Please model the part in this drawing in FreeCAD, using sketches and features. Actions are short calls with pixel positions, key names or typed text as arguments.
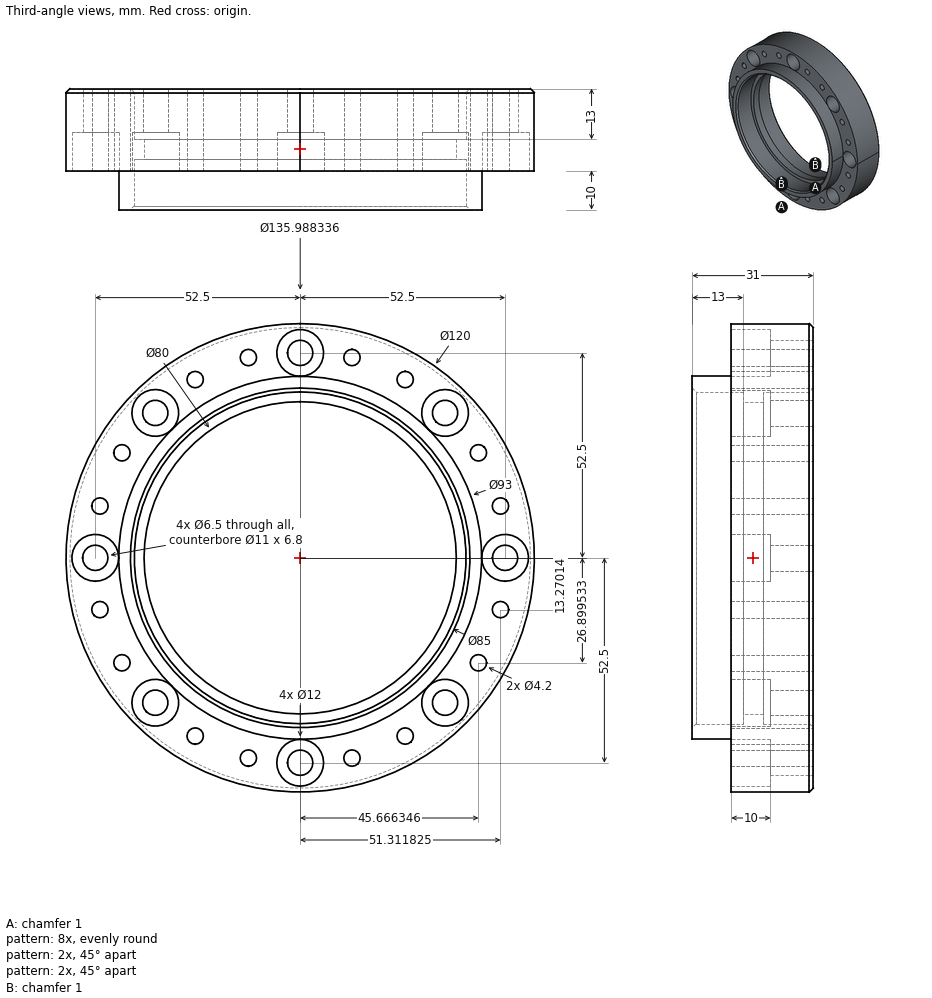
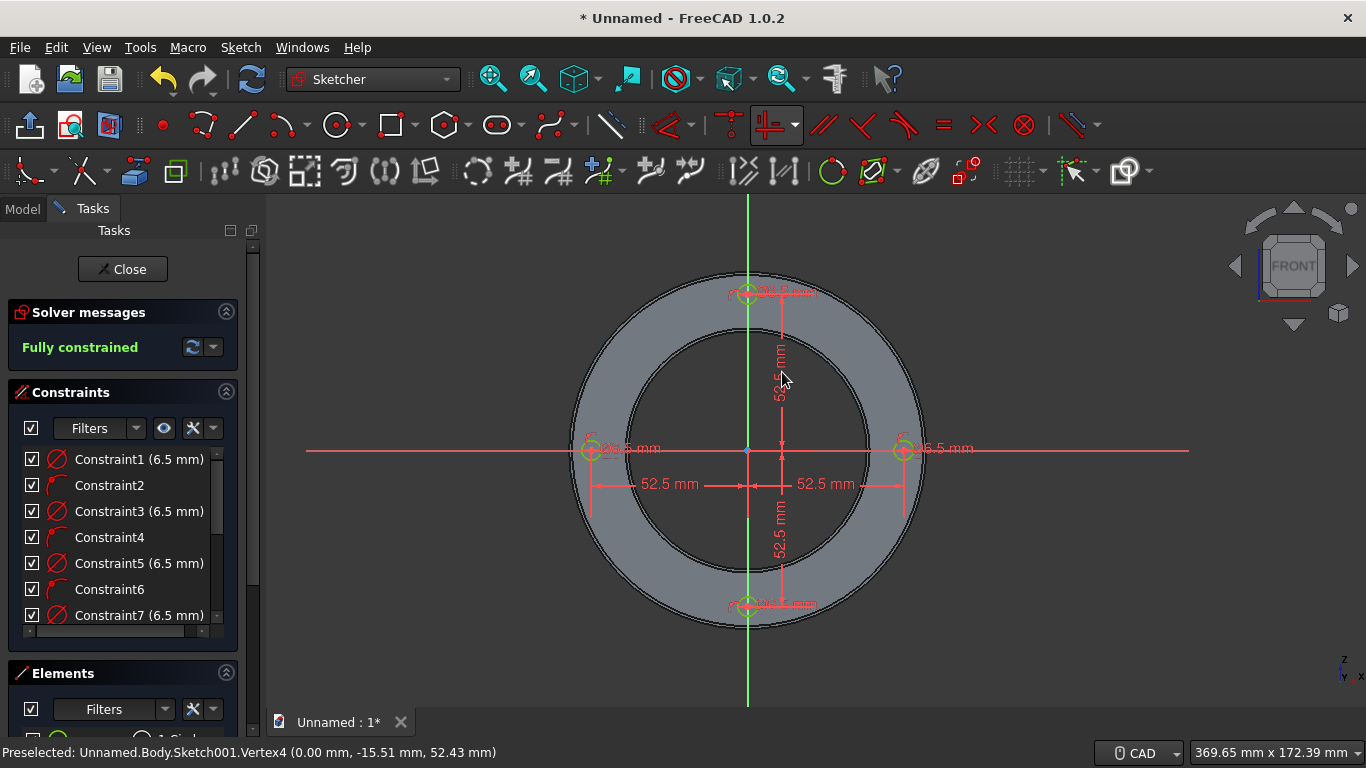
click(123, 269)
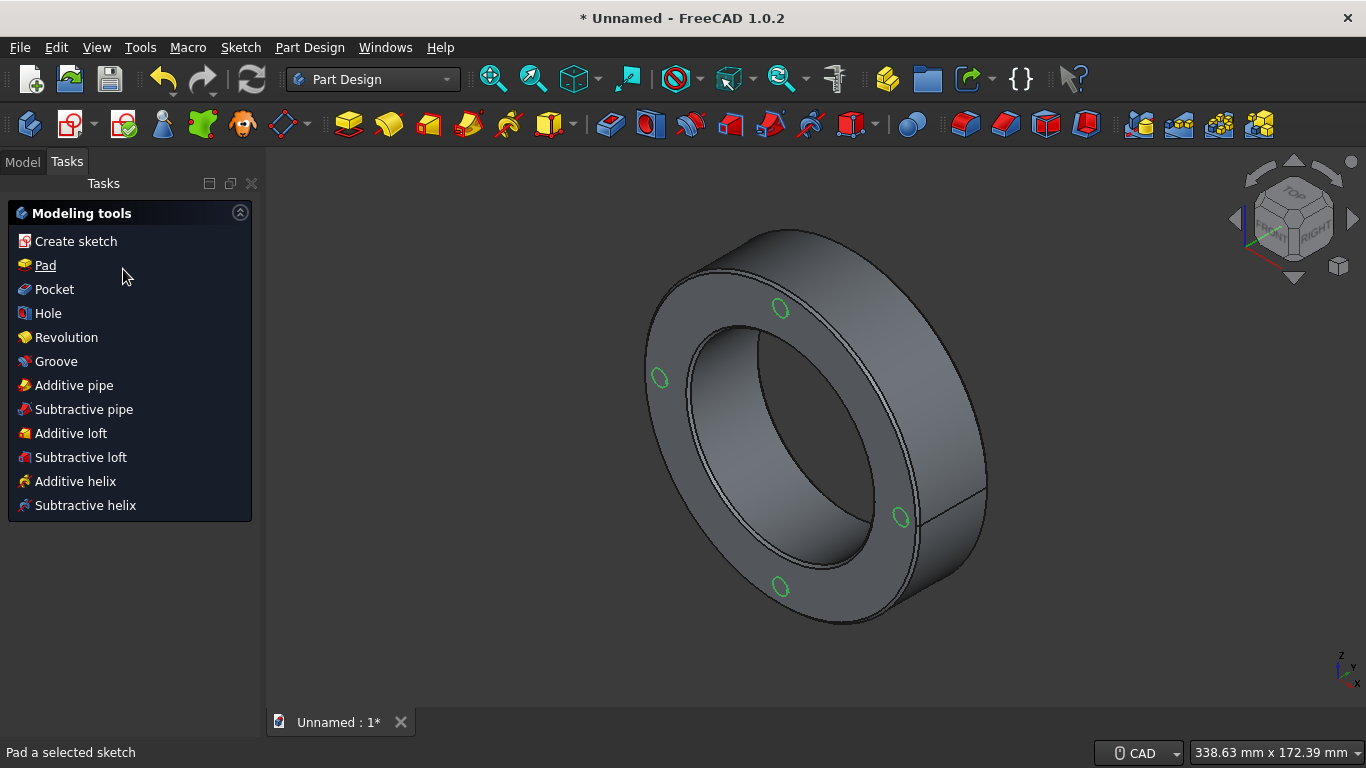
click(652, 124)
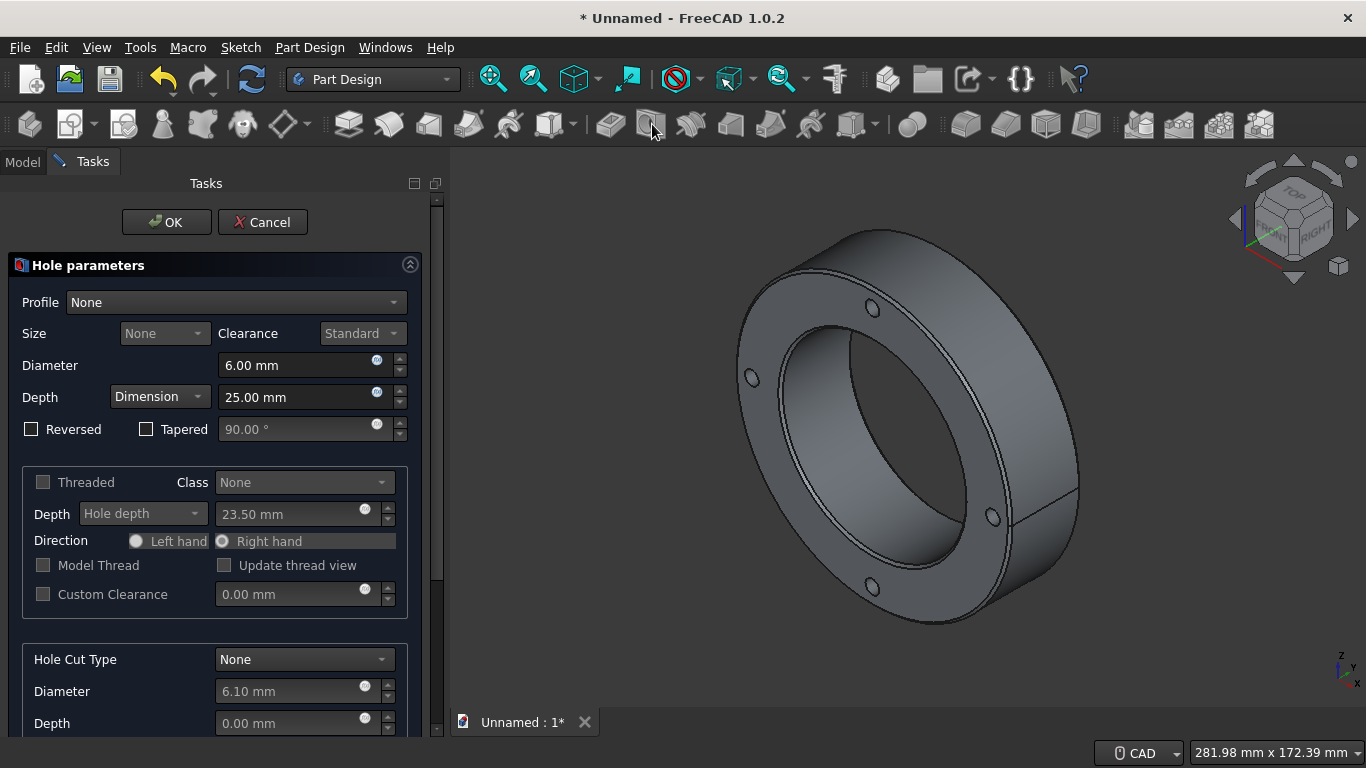
triple_click(305, 365)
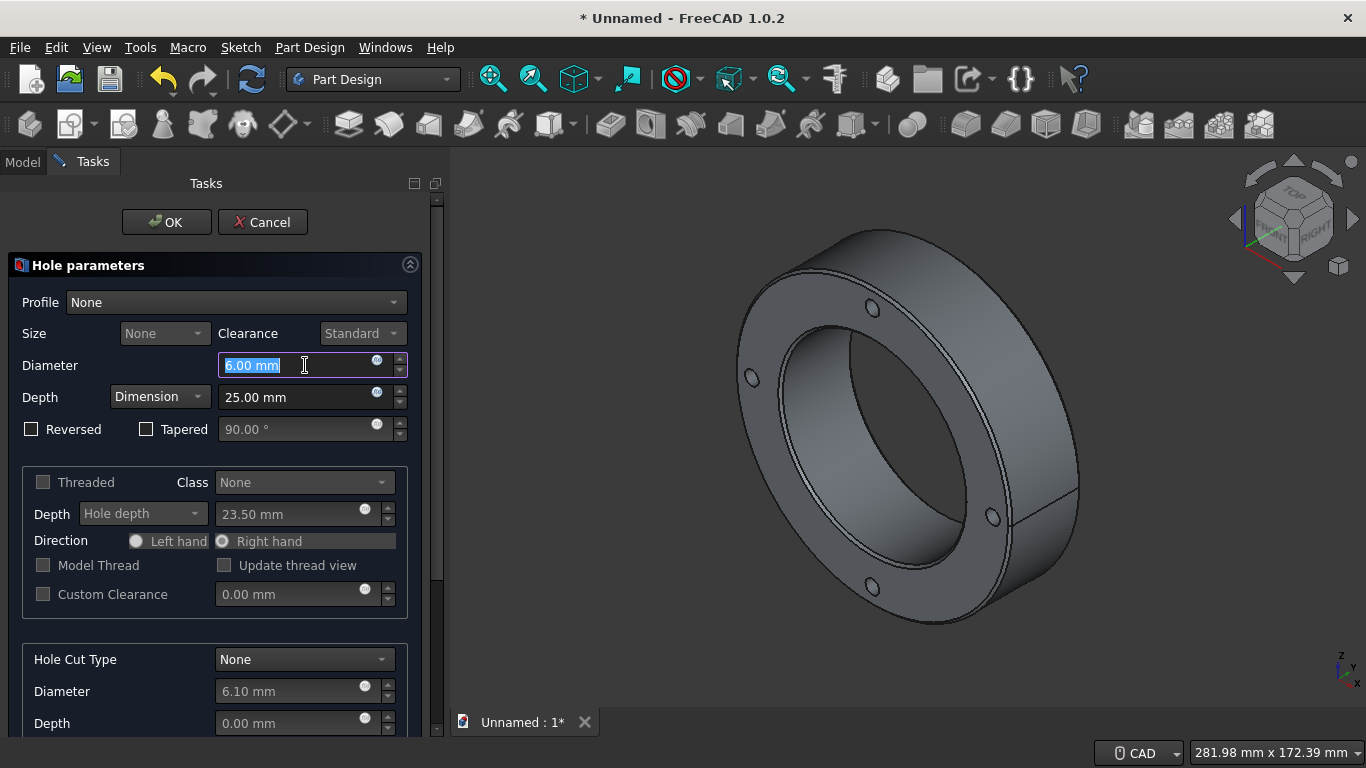
text(6.5)
key(Tab)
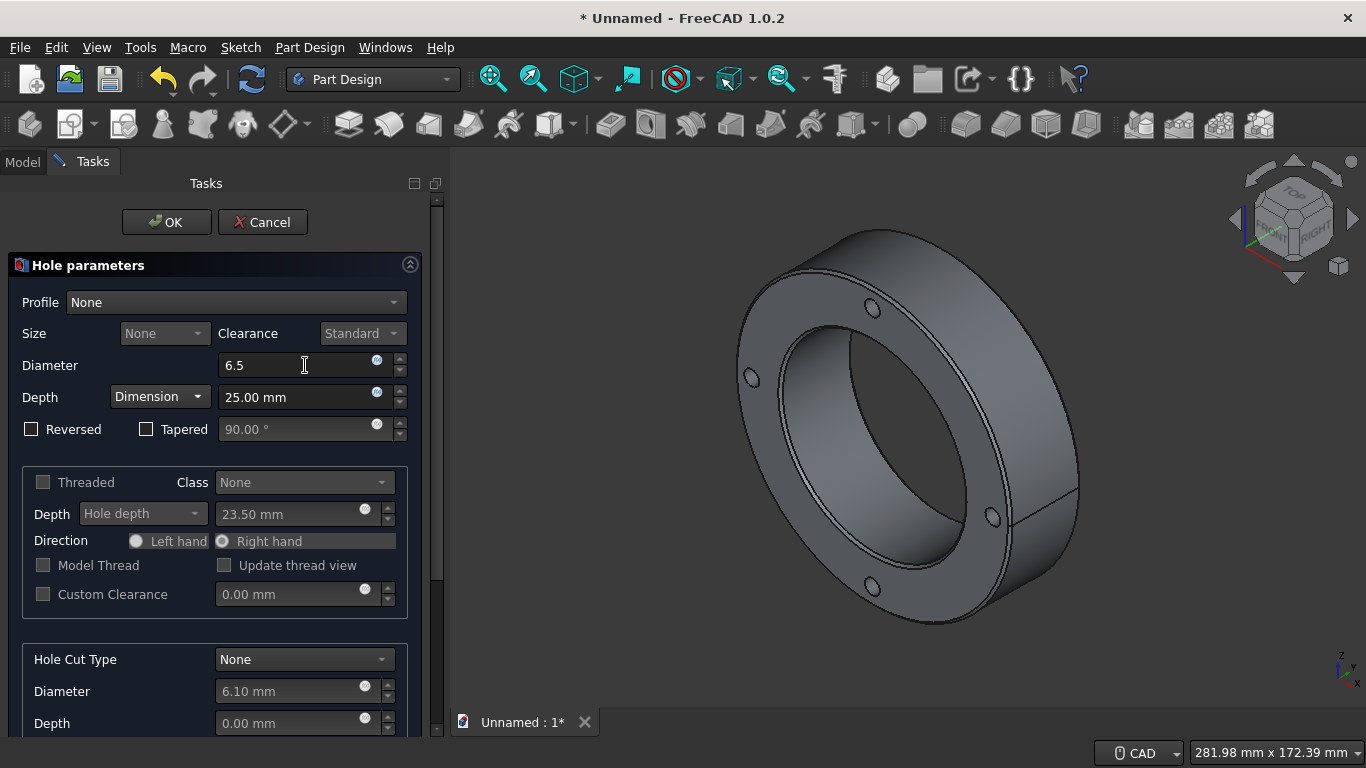
click(161, 396)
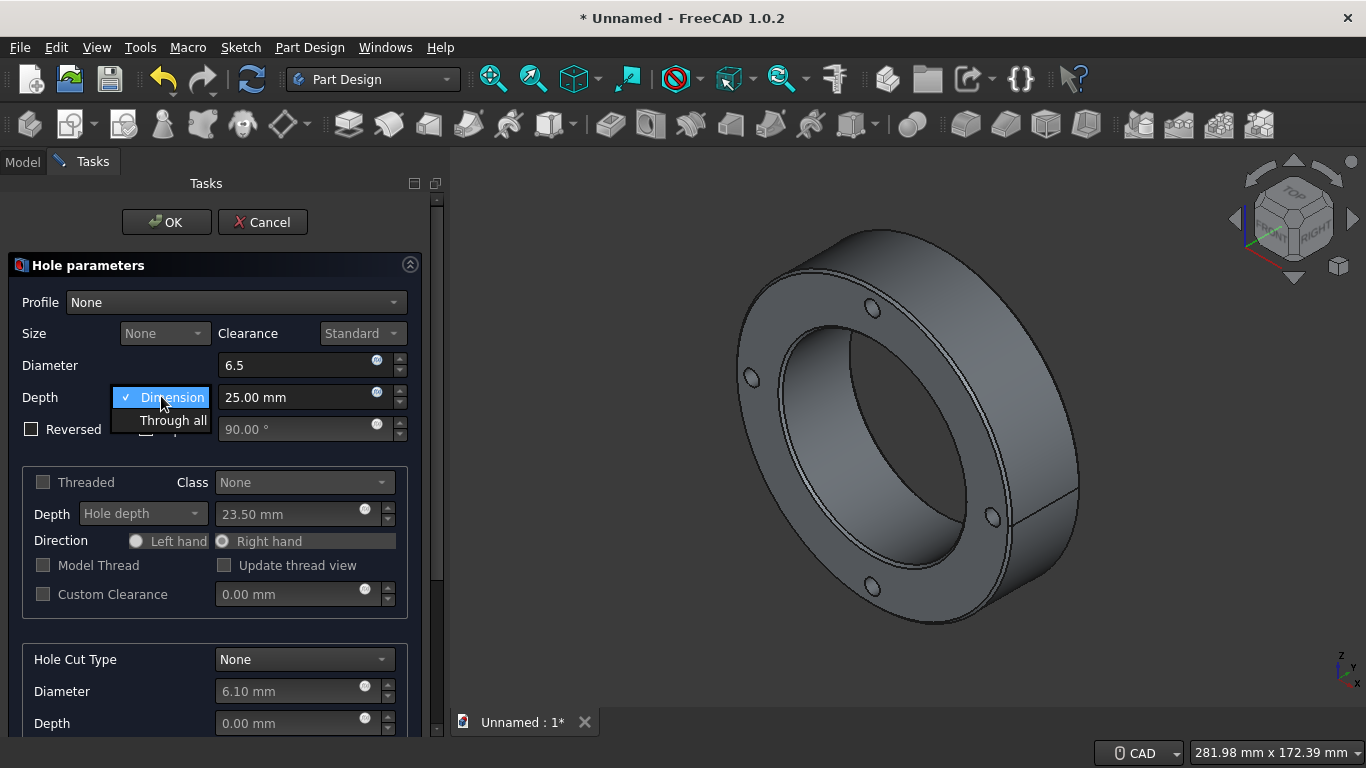
click(160, 420)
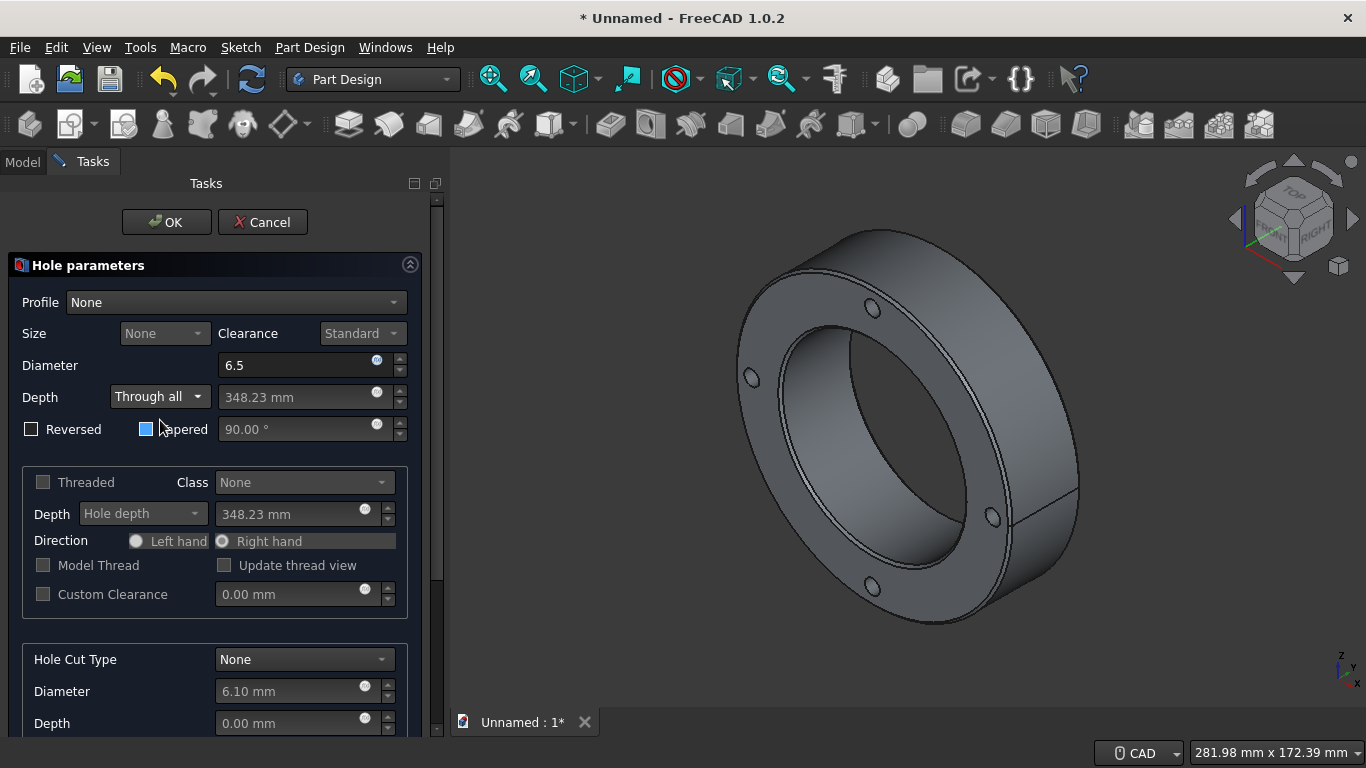
click(306, 660)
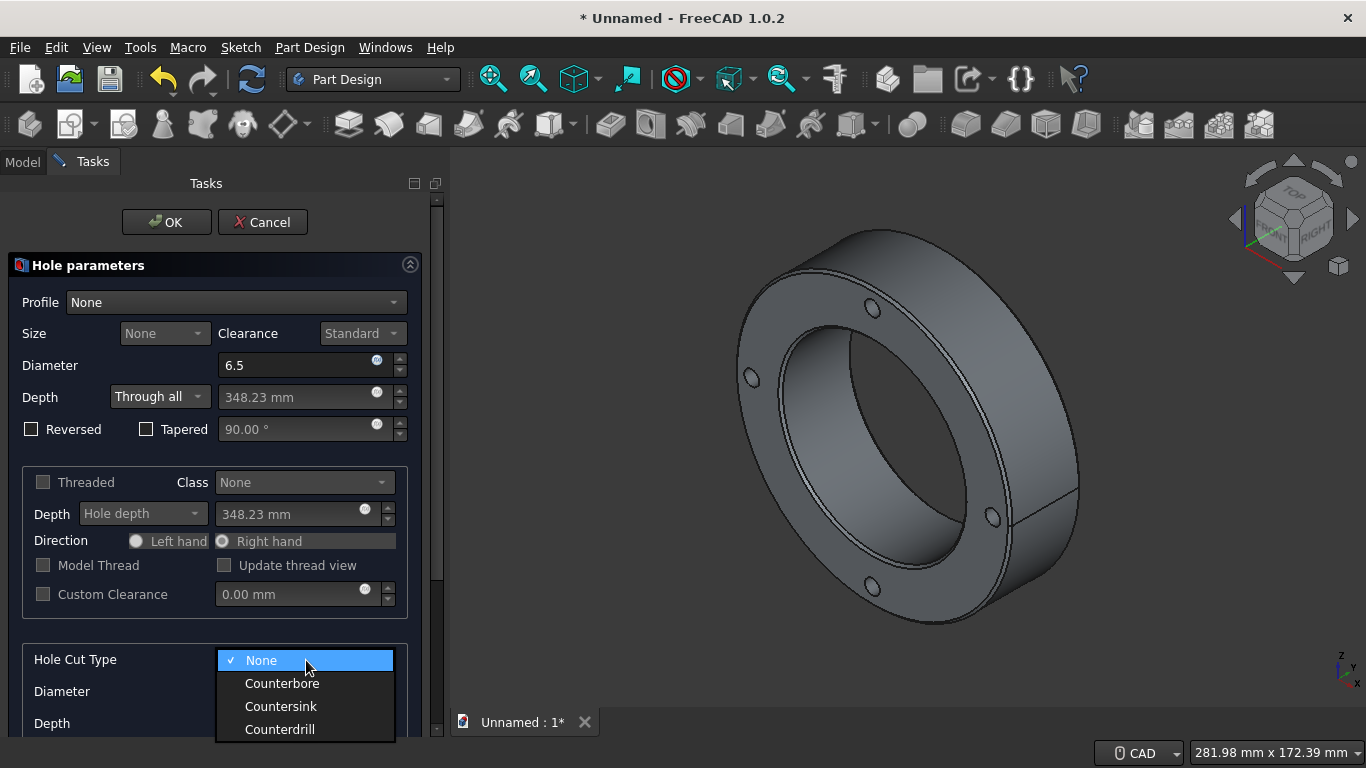
click(304, 684)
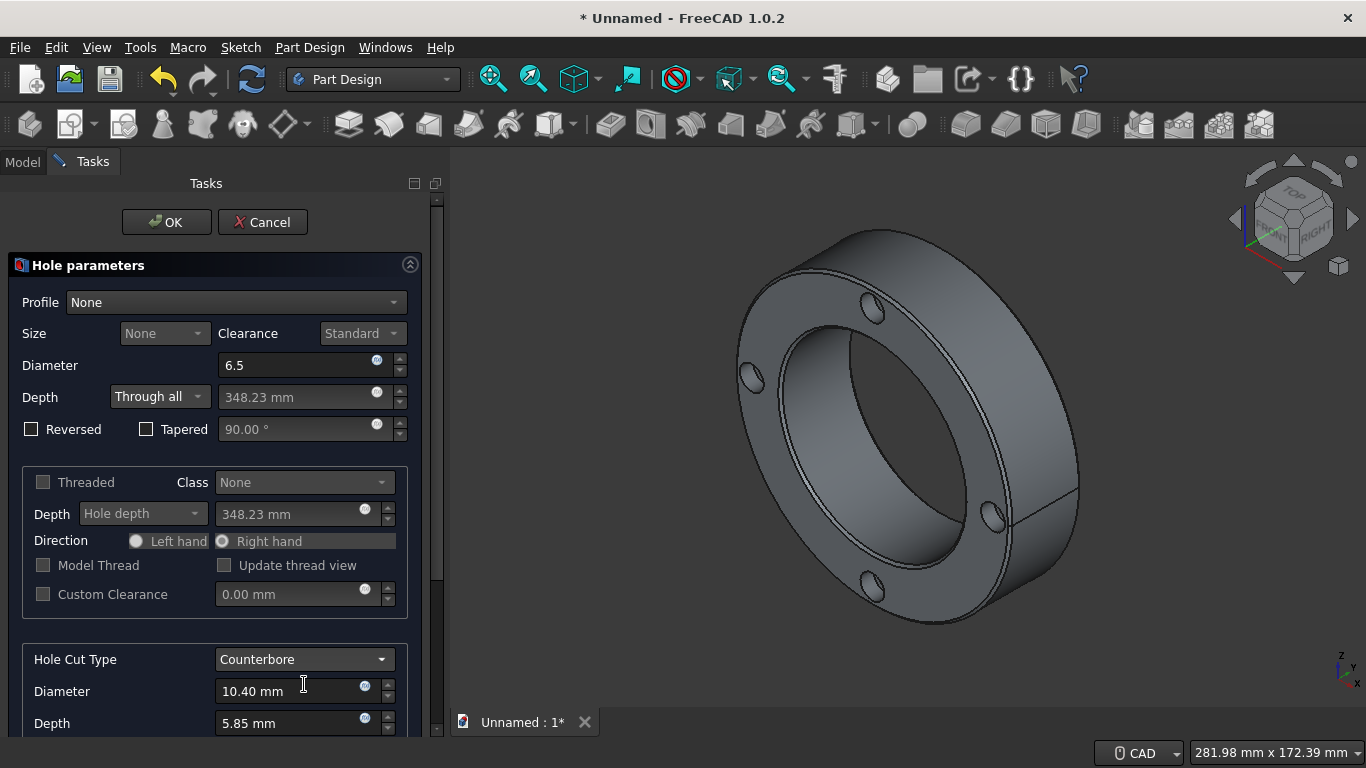
triple_click(298, 691)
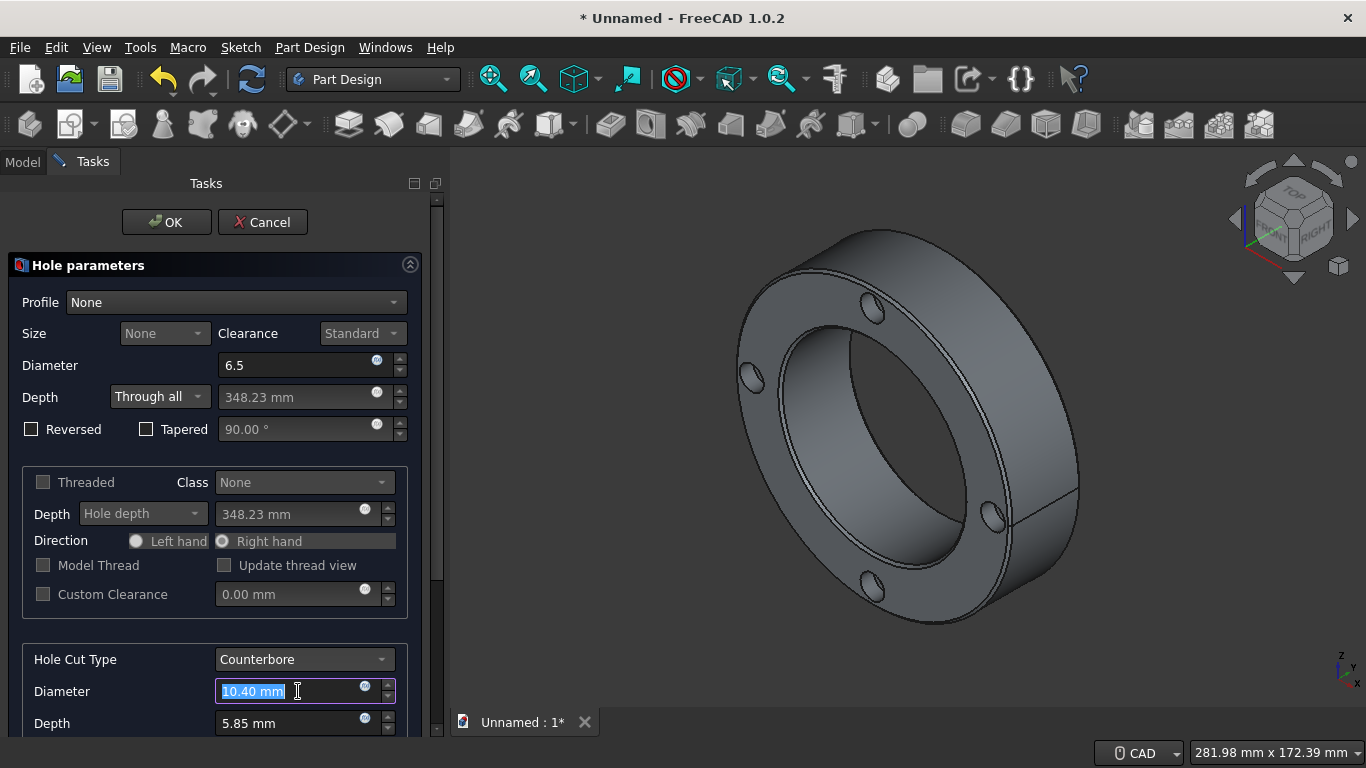
text(11)
key(Tab)